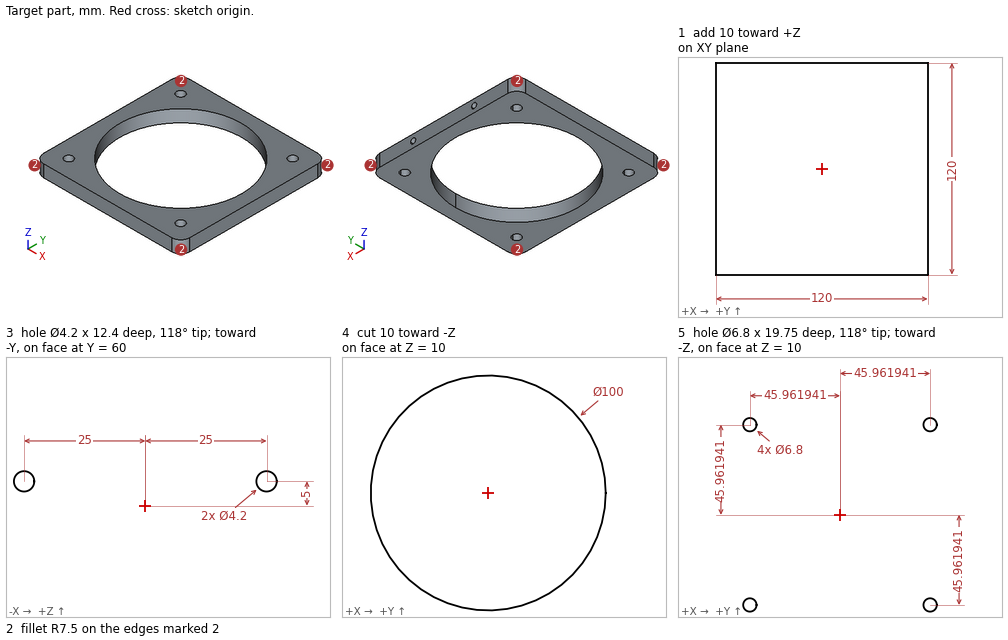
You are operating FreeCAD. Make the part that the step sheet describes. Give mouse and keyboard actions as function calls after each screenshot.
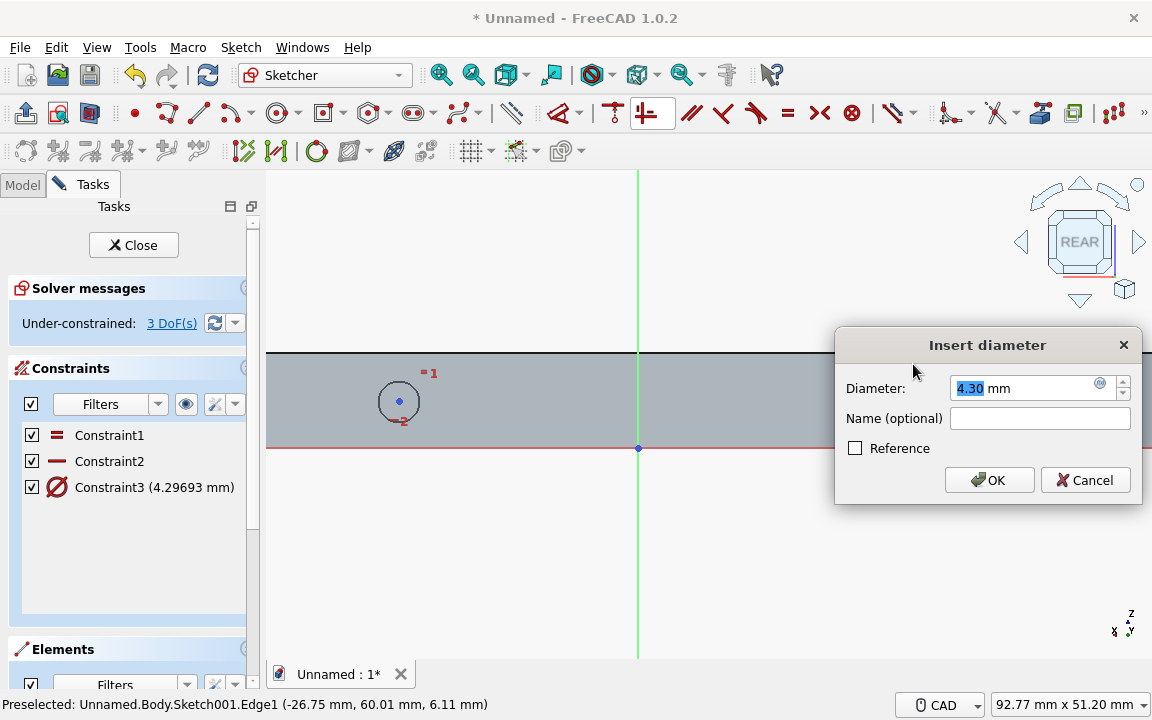
text(4.2)
key(Return)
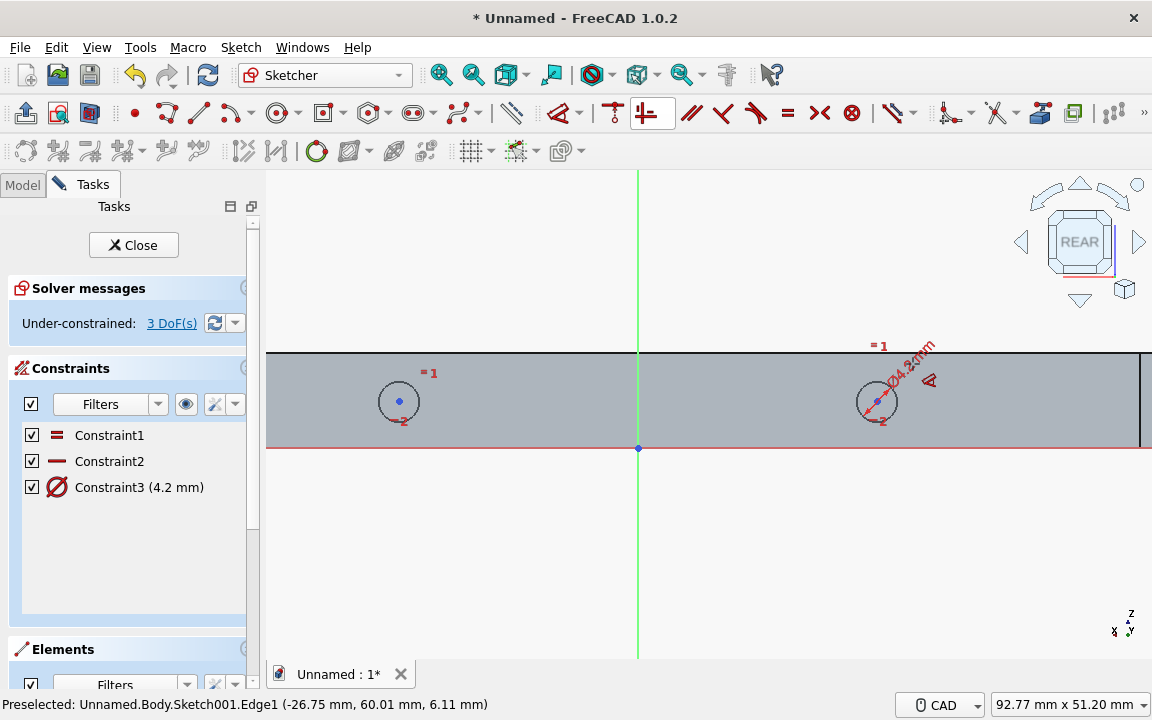
click(877, 402)
click(911, 425)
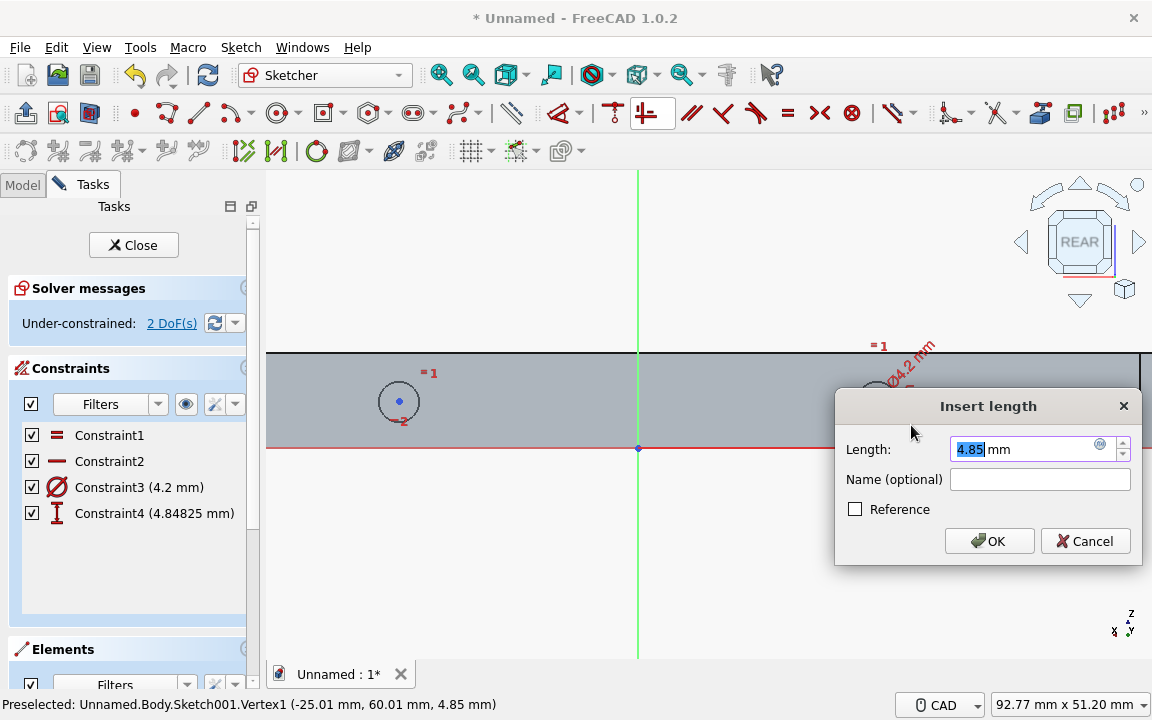
text(5)
key(Return)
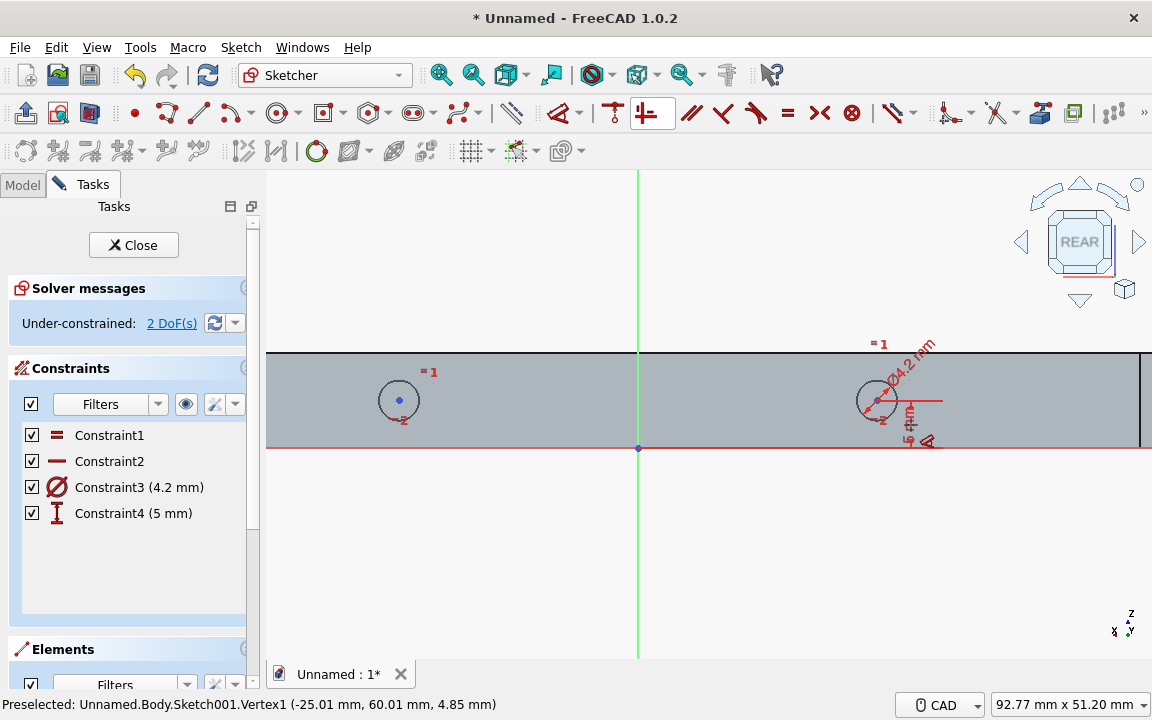
click(877, 401)
click(758, 482)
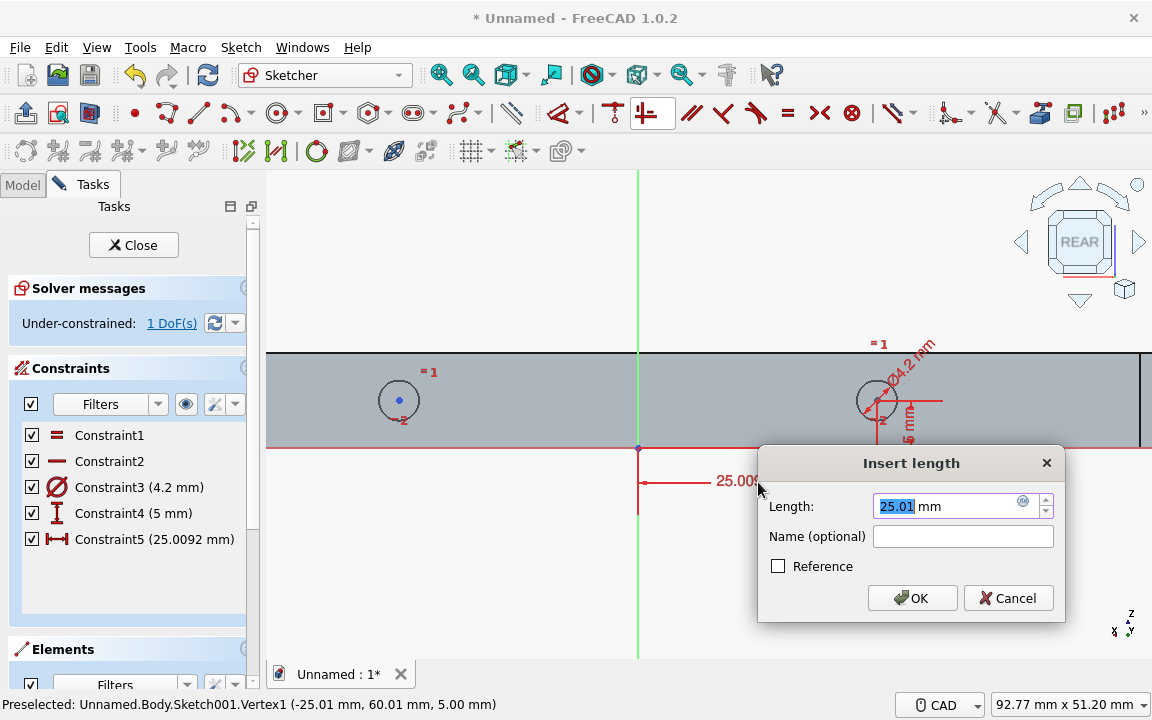
text(25)
key(Return)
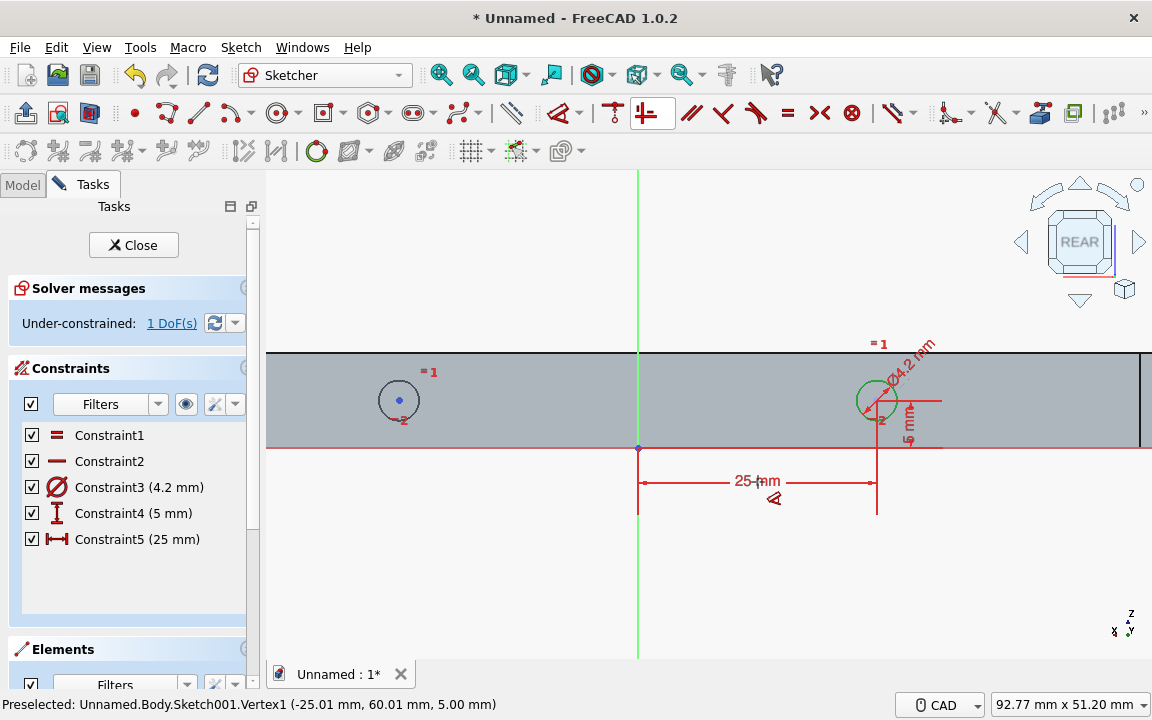
click(399, 401)
click(519, 482)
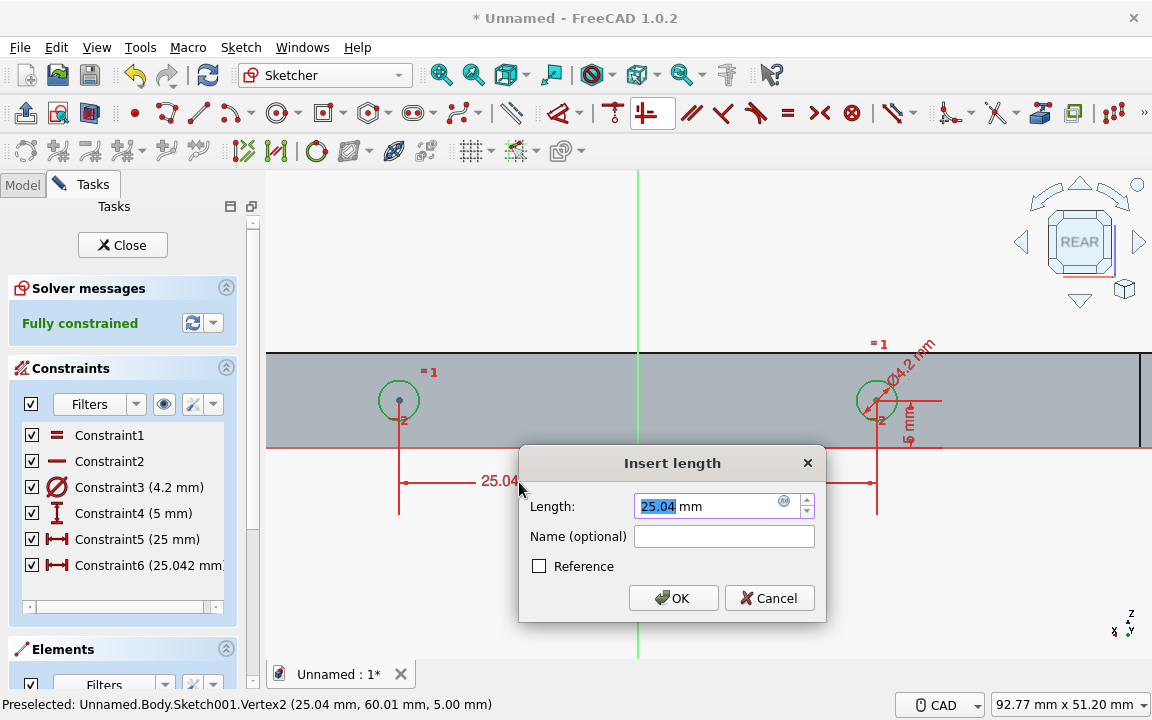
text(25)
key(Return)
key(Escape)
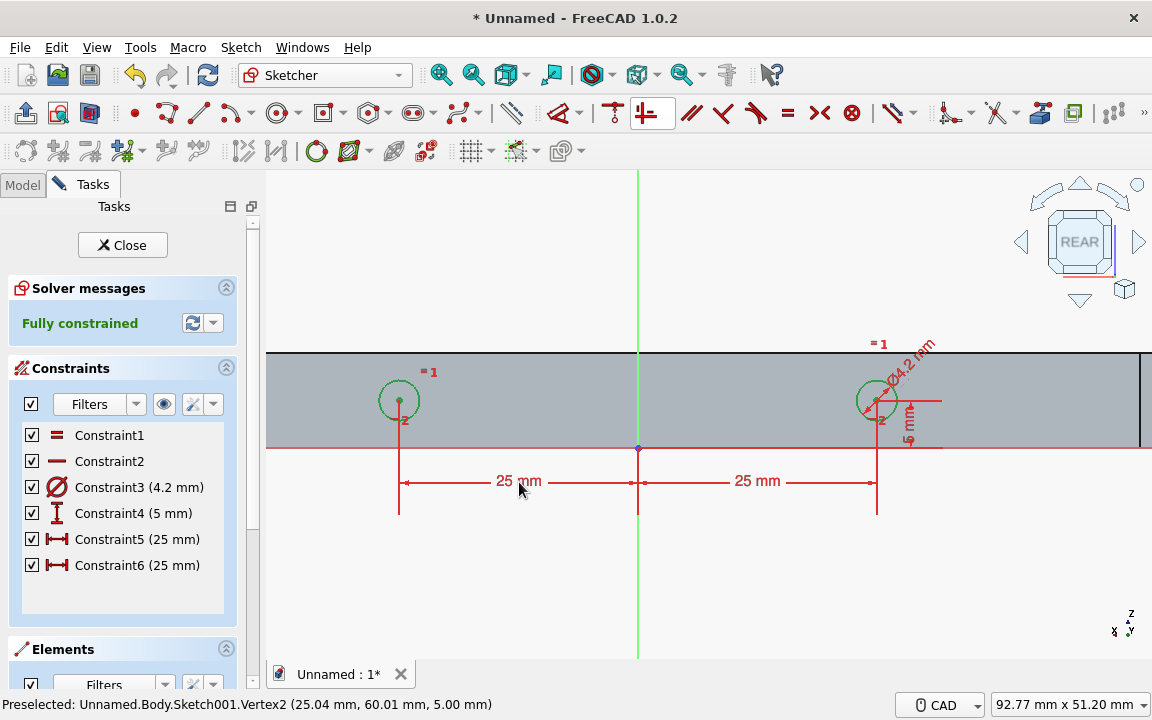
click(123, 245)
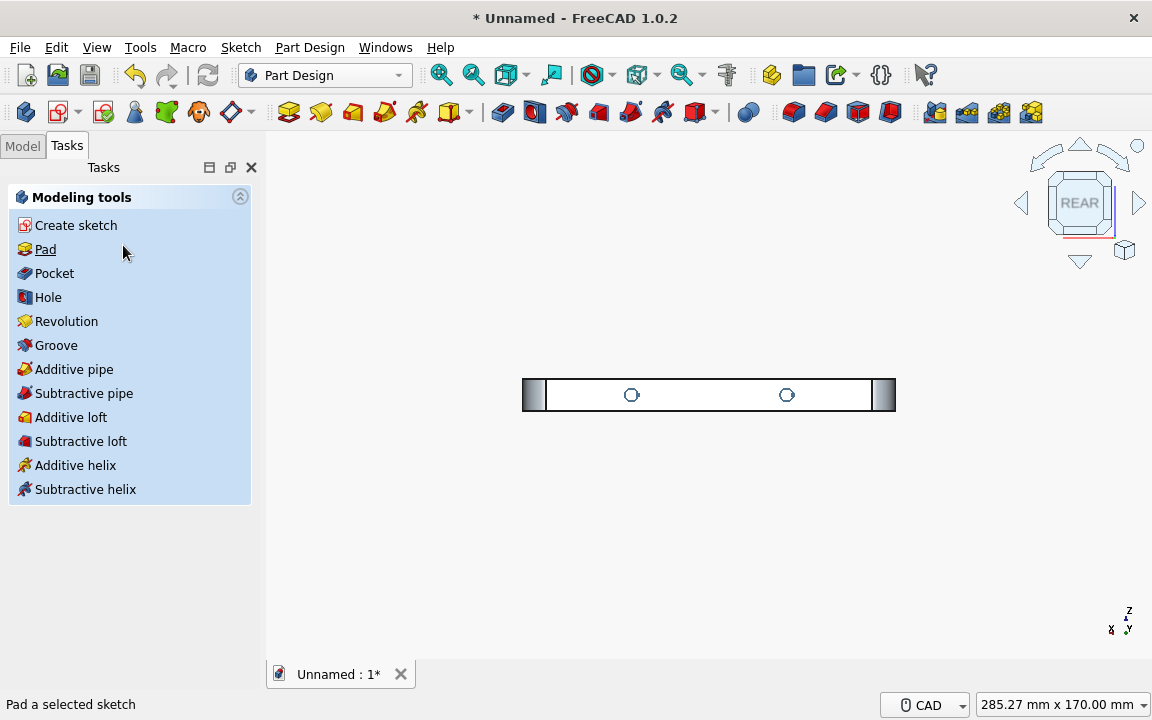
click(536, 112)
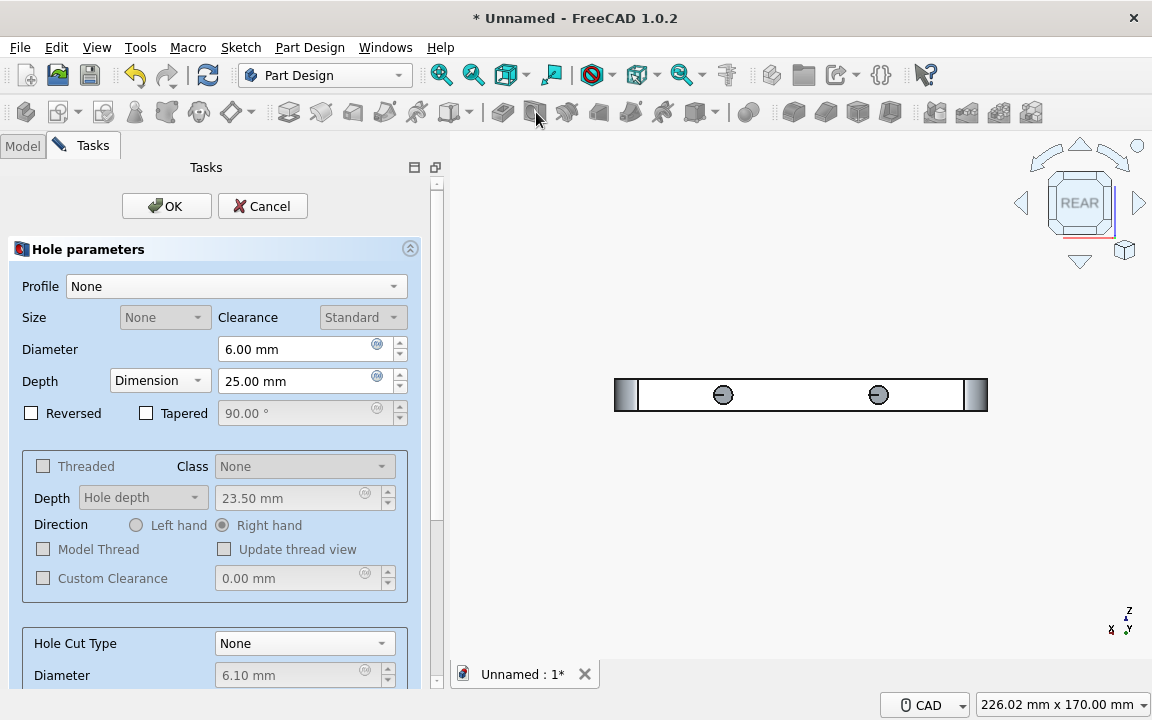
triple_click(305, 349)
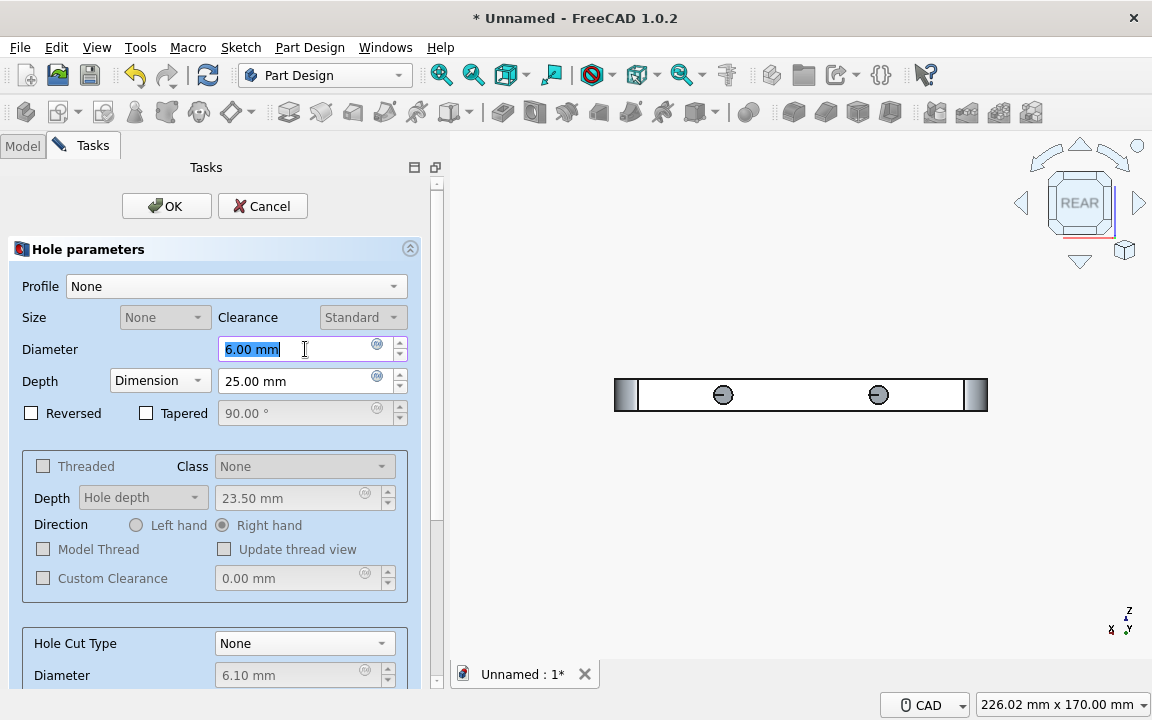
text(4.2)
key(Tab)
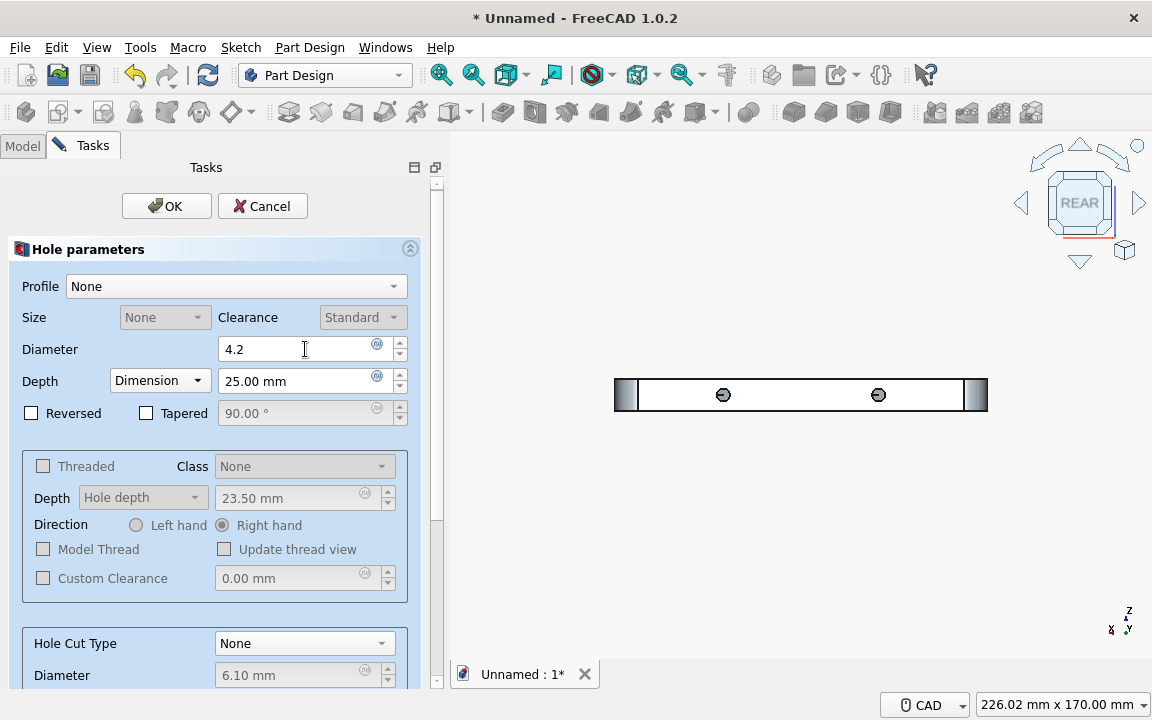
triple_click(305, 381)